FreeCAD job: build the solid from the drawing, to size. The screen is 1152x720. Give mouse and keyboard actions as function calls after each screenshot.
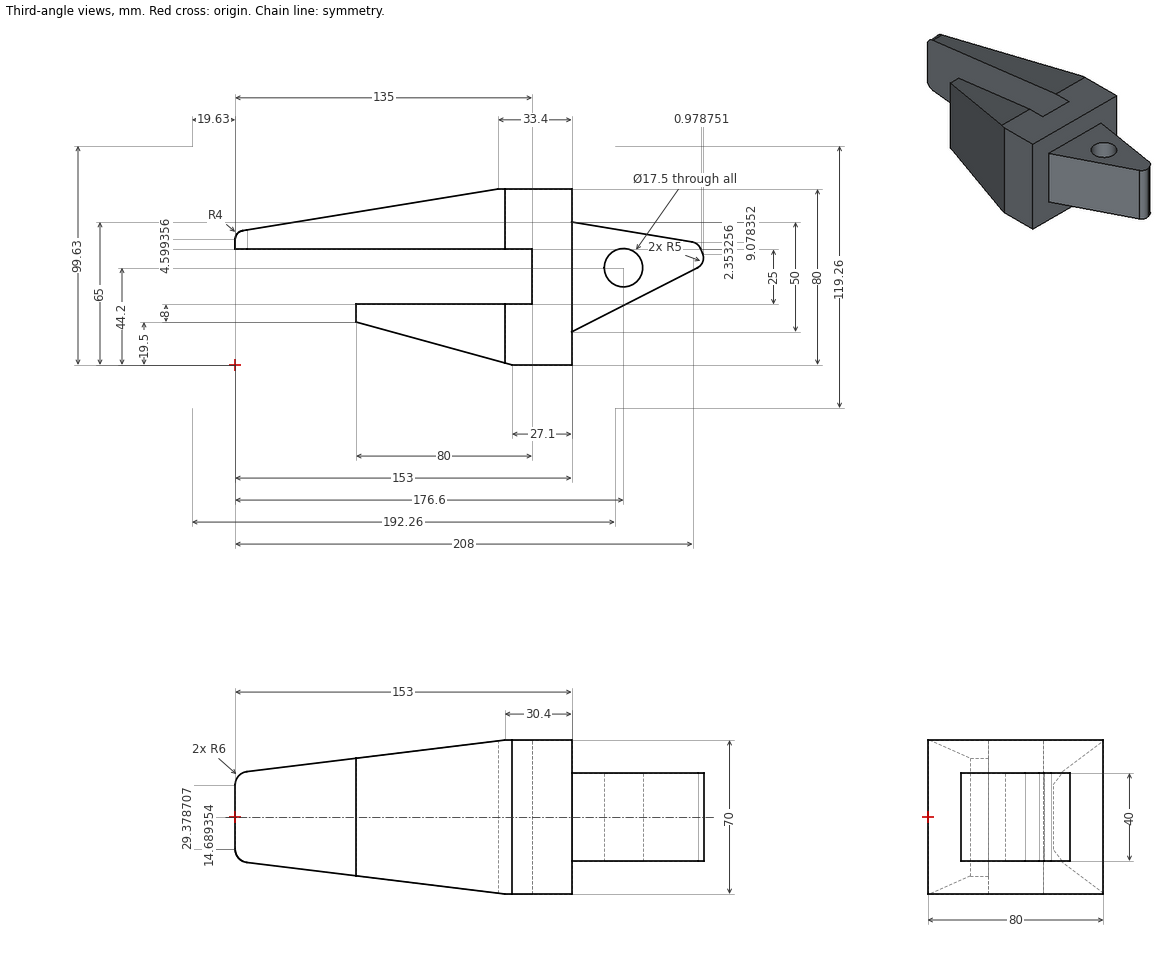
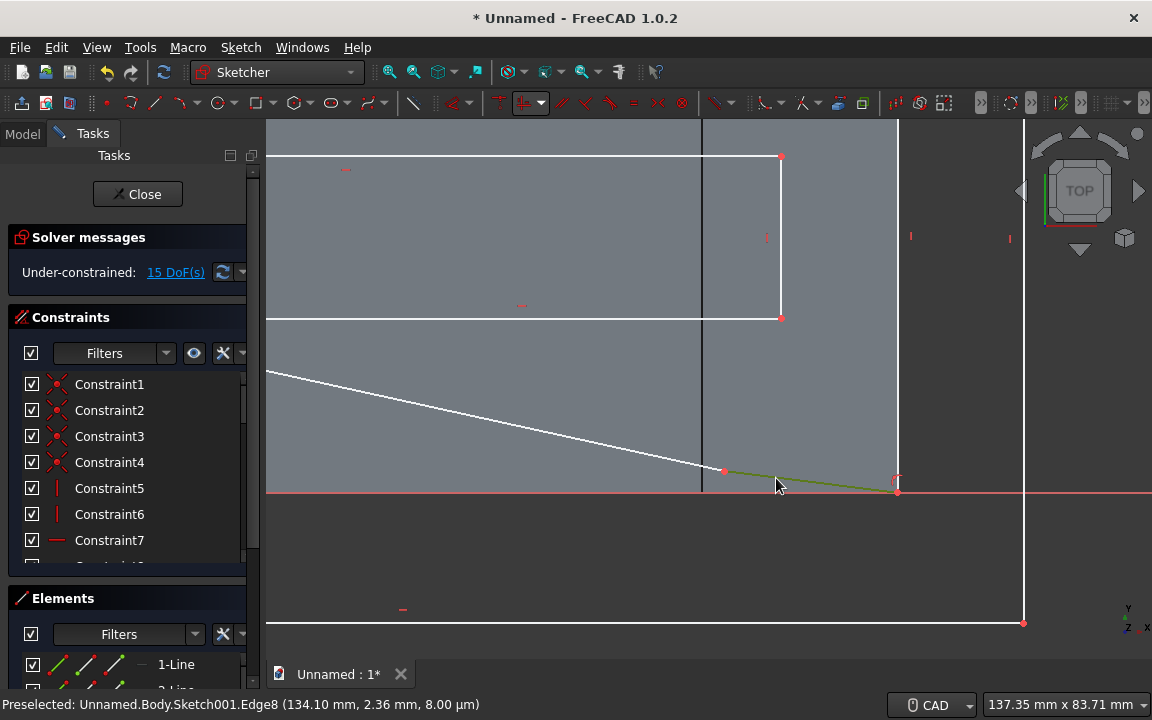
key(h)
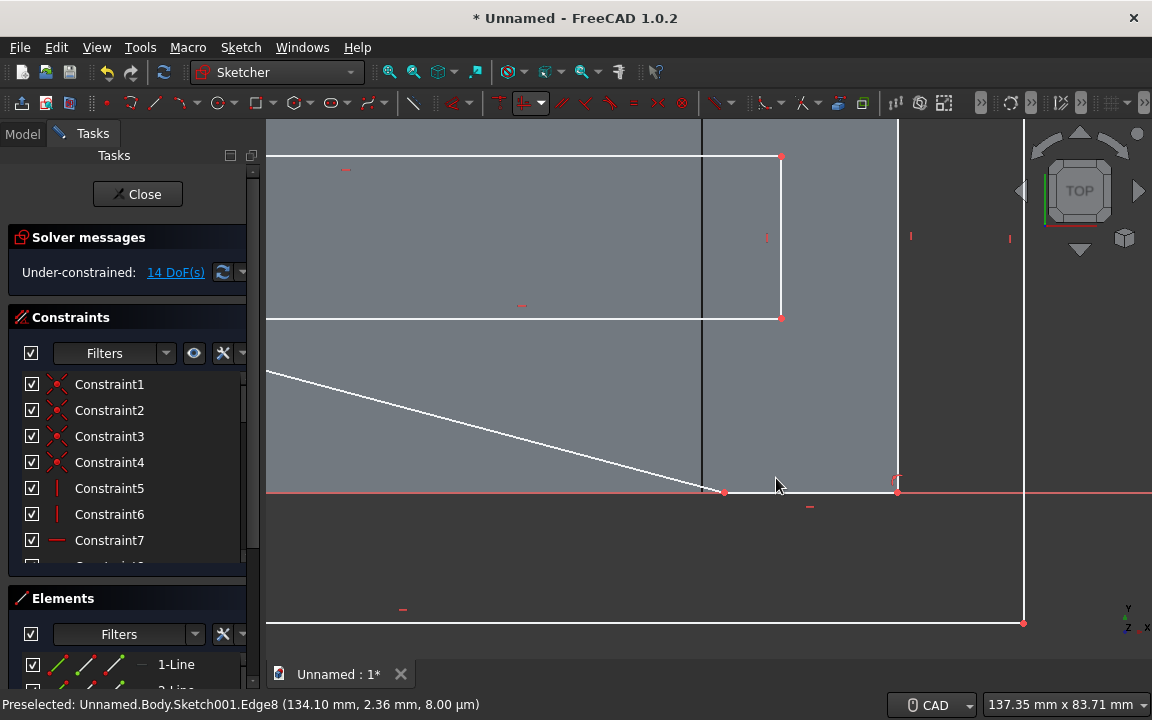
scroll(778, 479, down, 5)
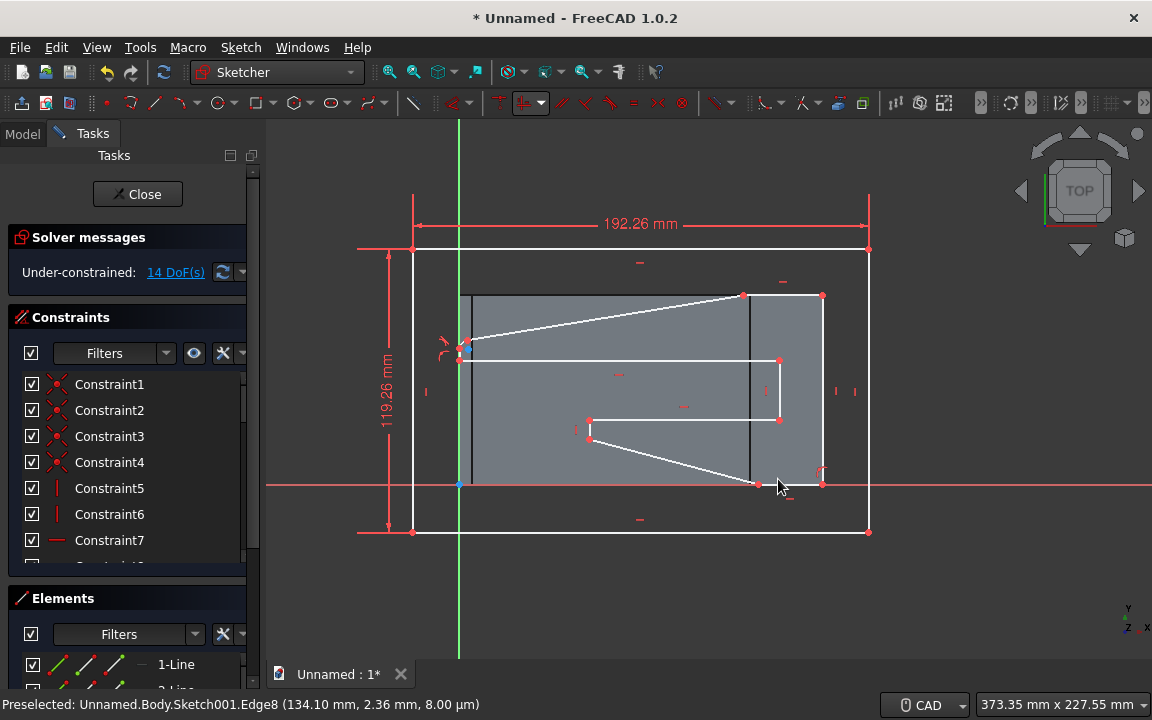
scroll(460, 357, up, 7)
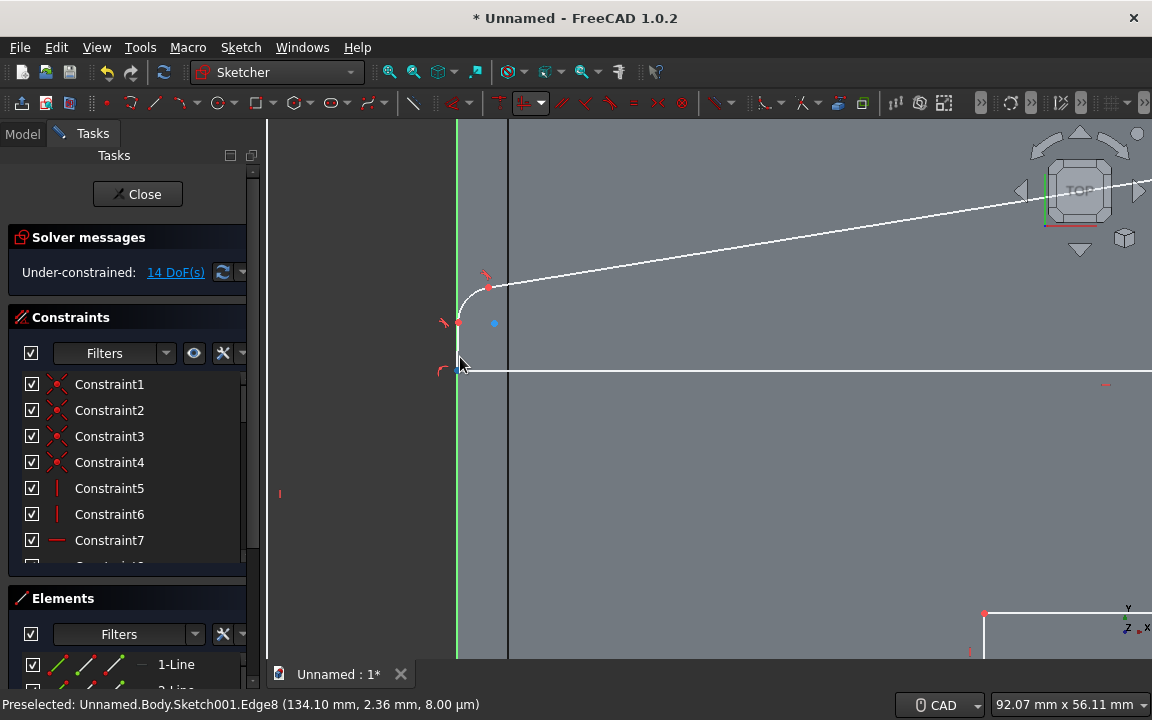
click(457, 356)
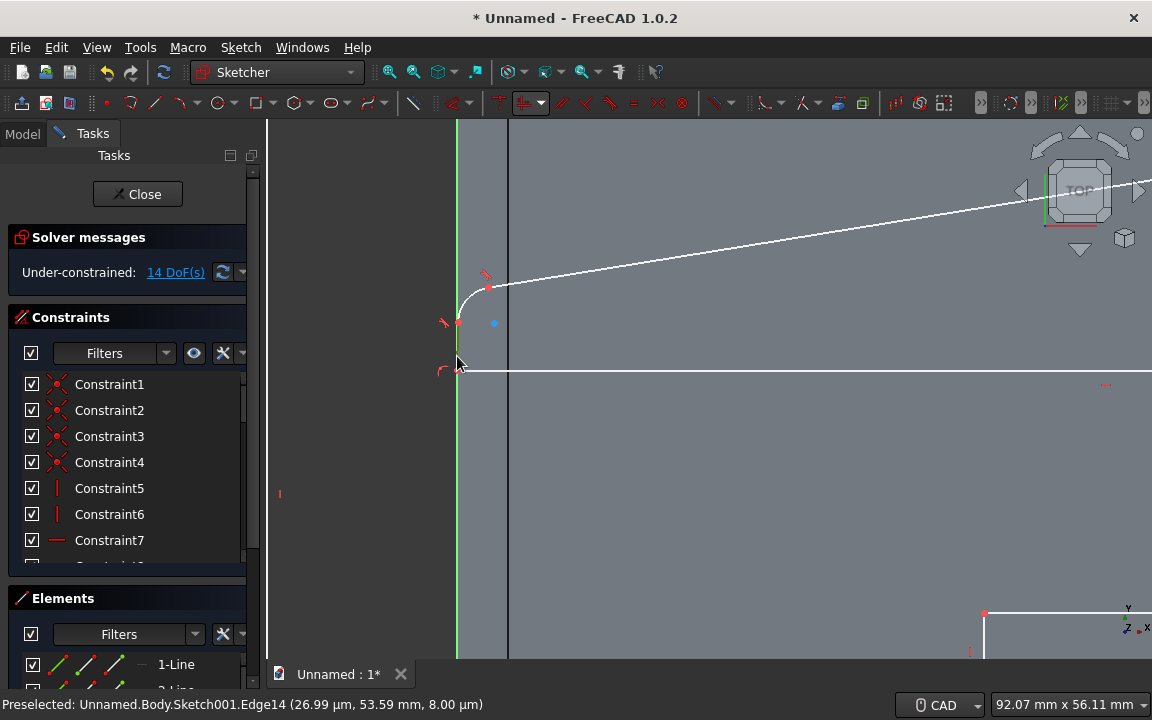
key(v)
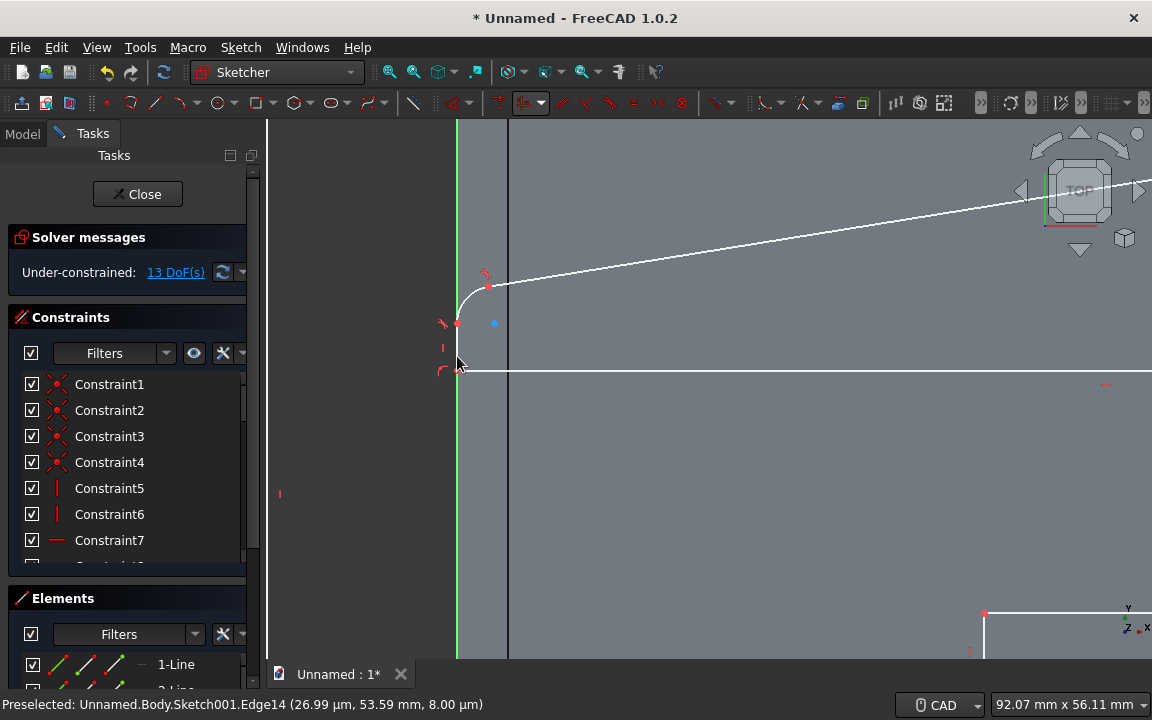
click(452, 104)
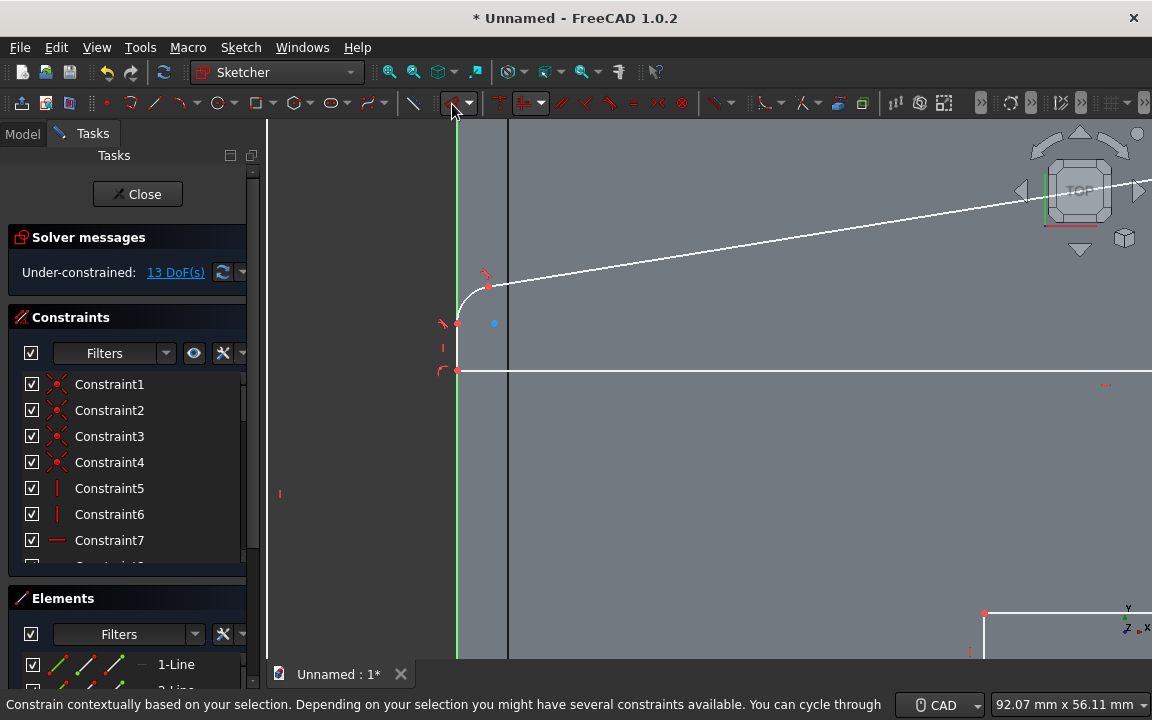
click(474, 292)
click(489, 254)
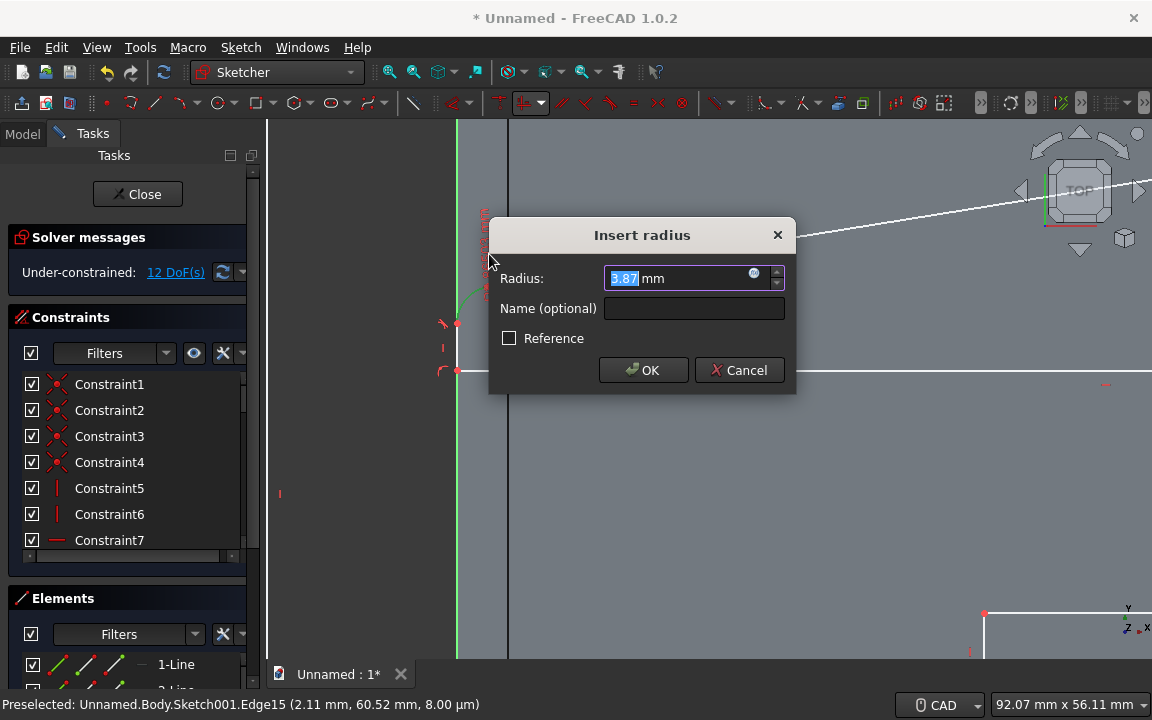
text(4)
key(Return)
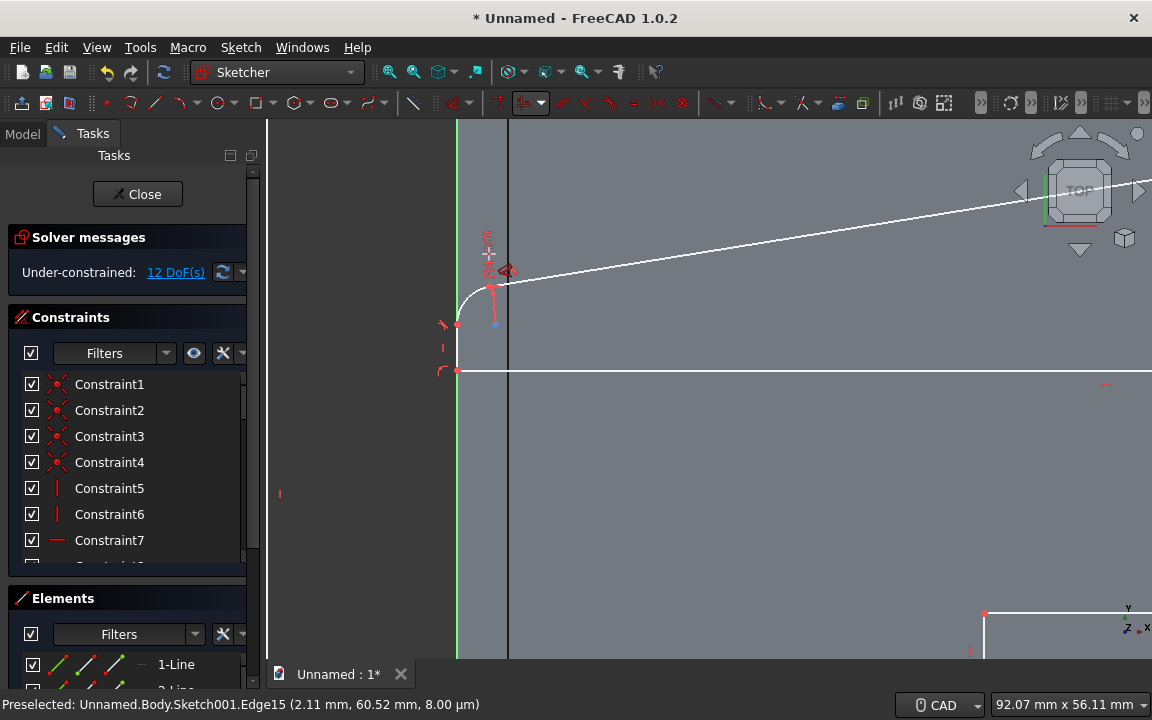
click(984, 629)
click(950, 622)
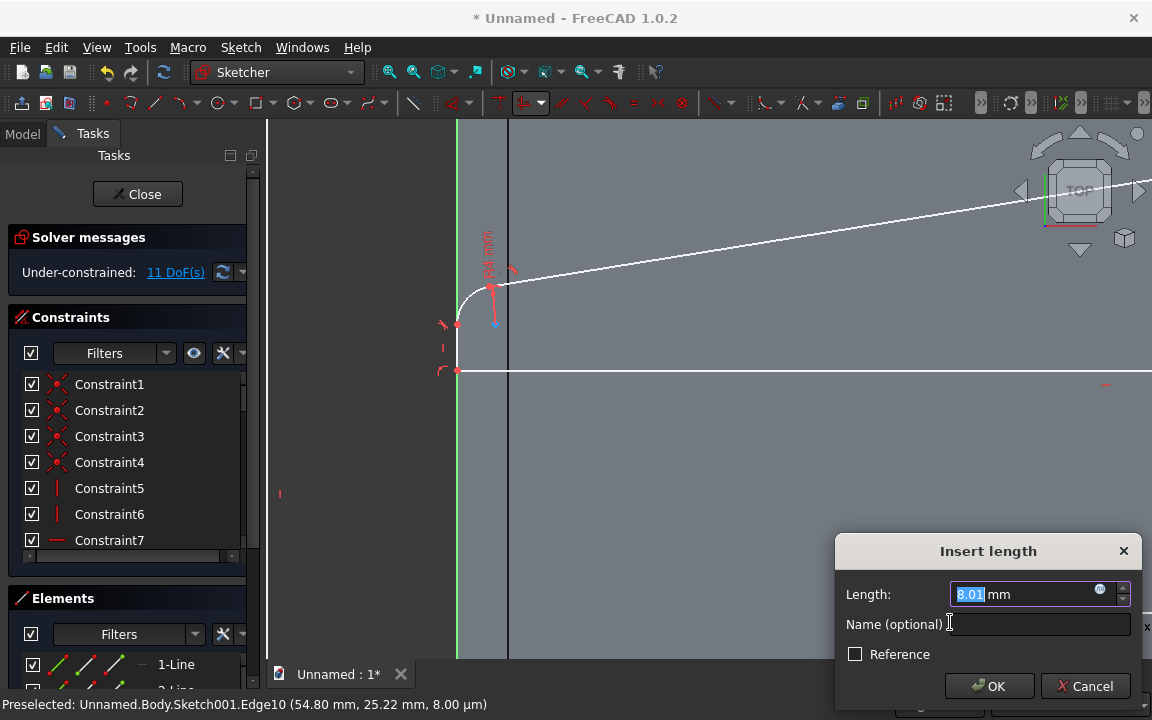
text(8)
key(Return)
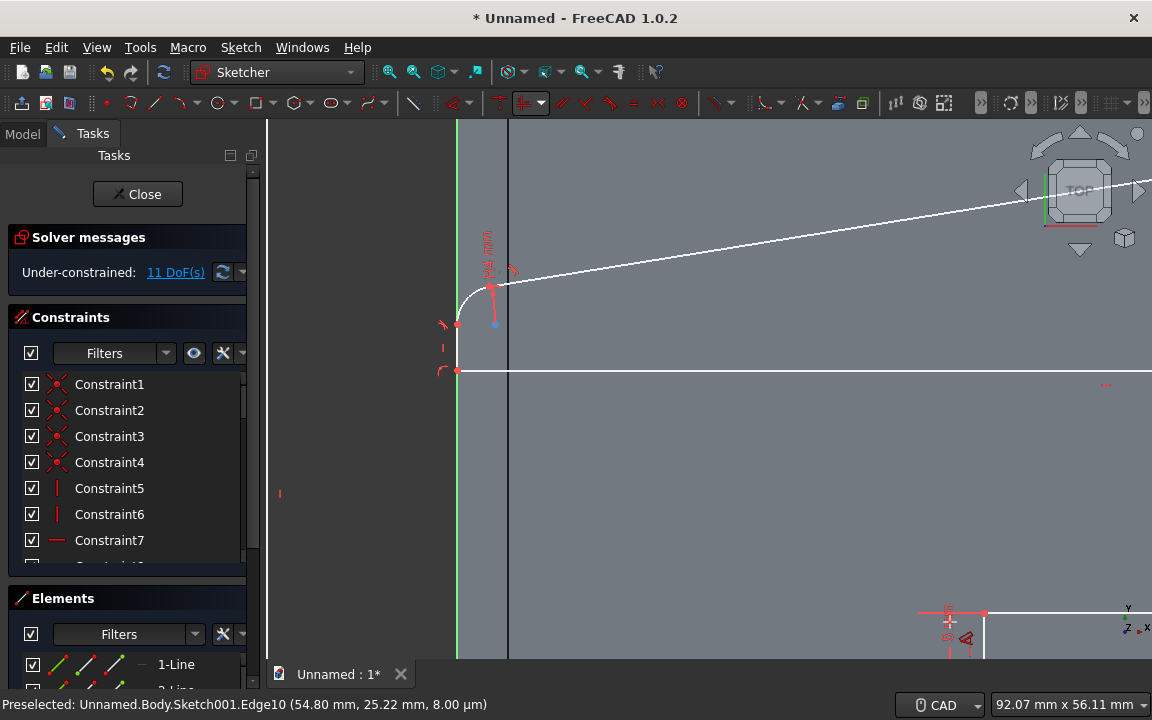
scroll(460, 357, down, 7)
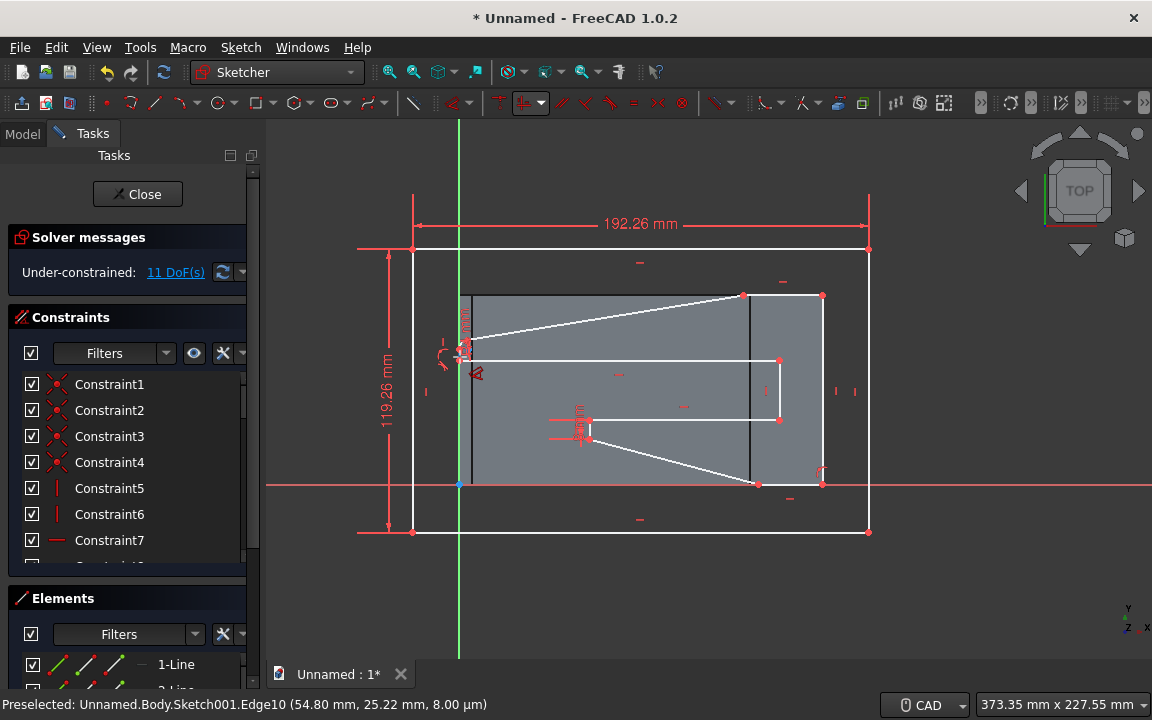
click(823, 352)
click(789, 347)